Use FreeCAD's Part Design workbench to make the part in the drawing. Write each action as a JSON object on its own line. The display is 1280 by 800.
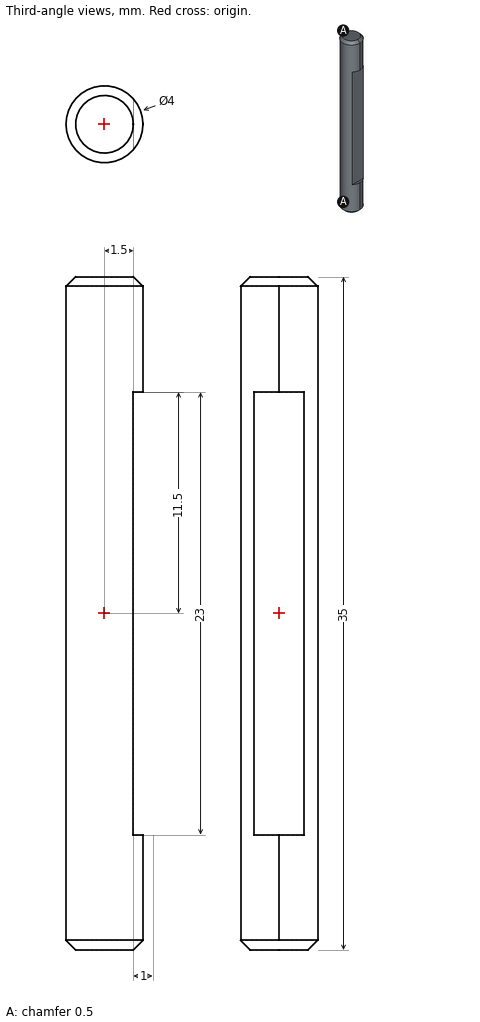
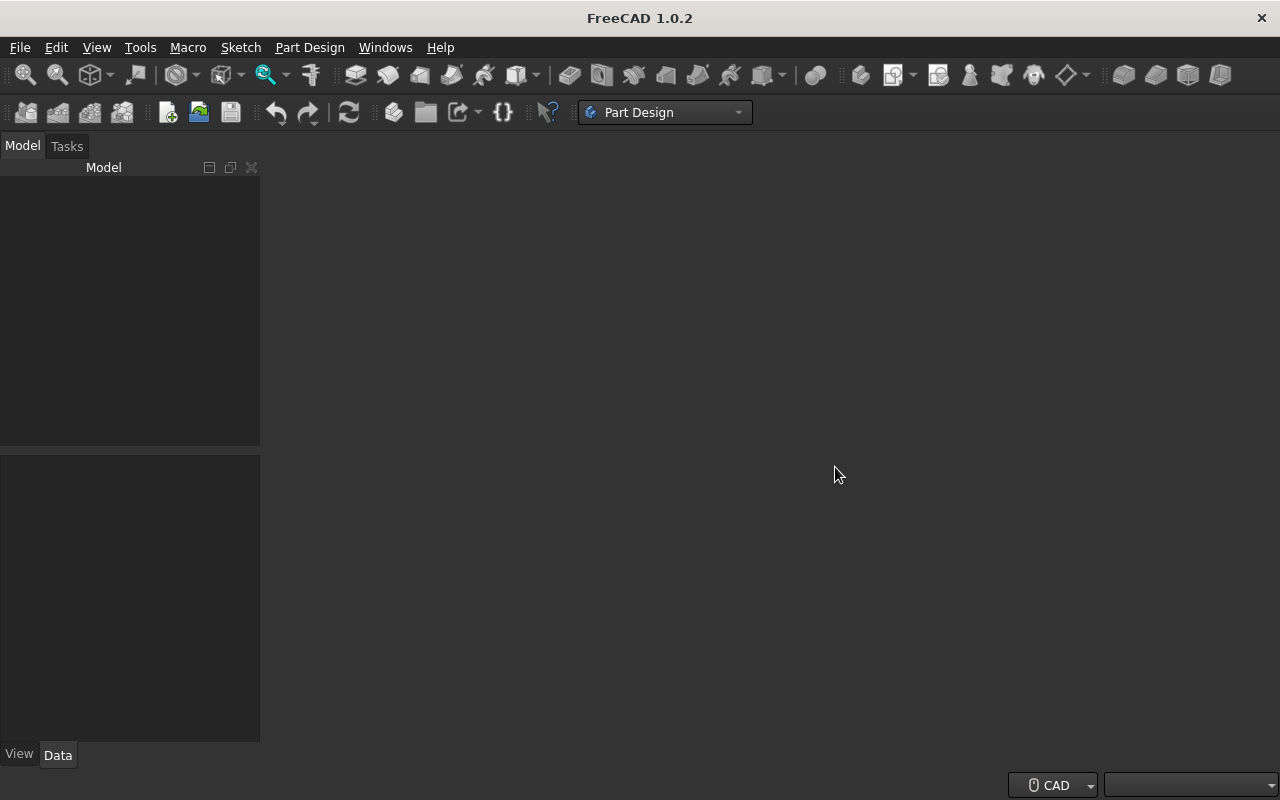
{"action": "left_click", "coordinate": [168, 112]}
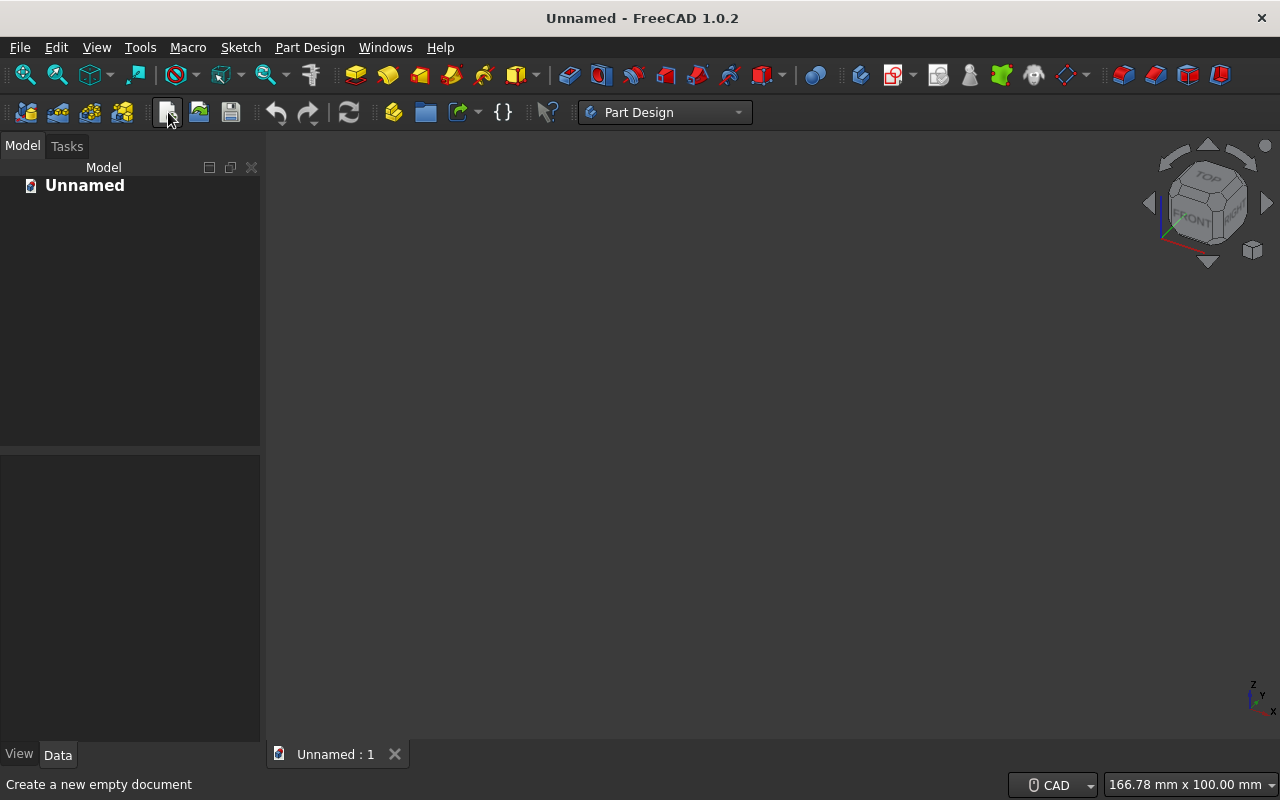
{"action": "left_click", "coordinate": [894, 76]}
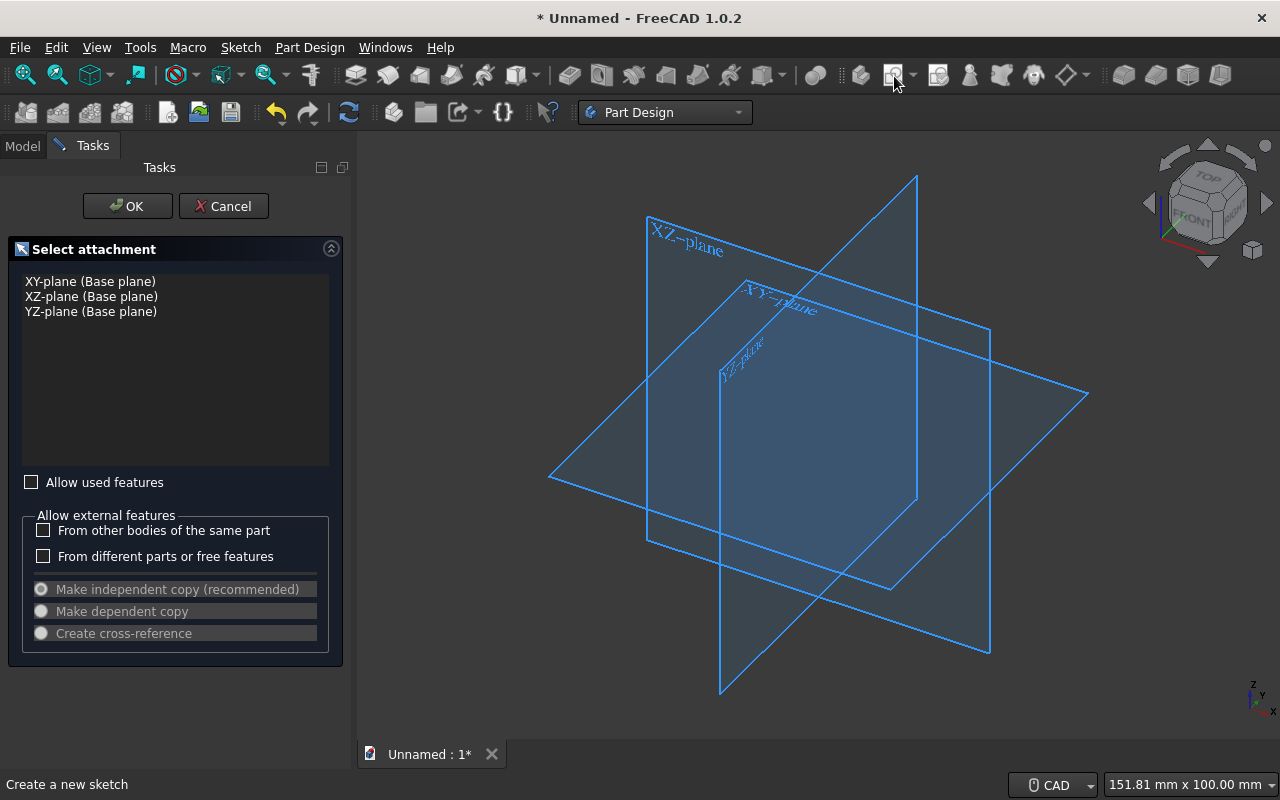
{"action": "left_click", "coordinate": [82, 282]}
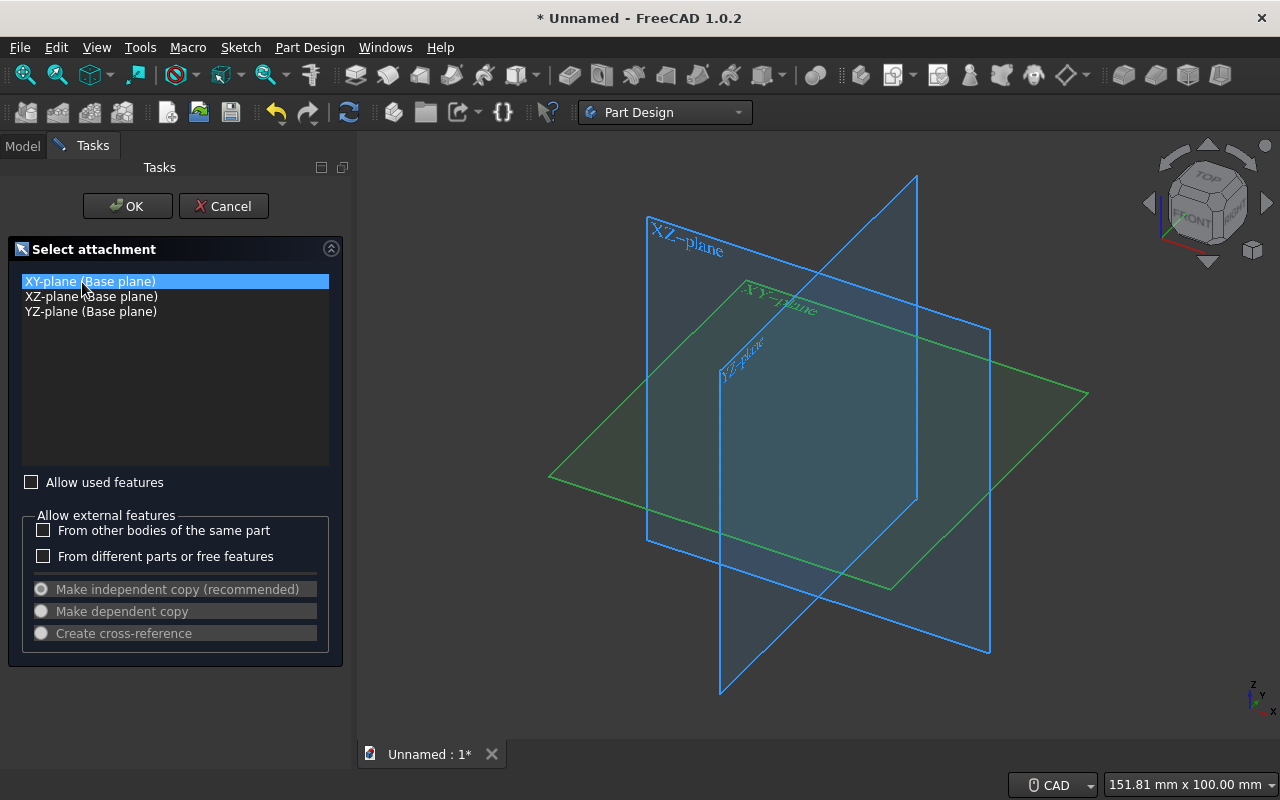
{"action": "left_click", "coordinate": [128, 206]}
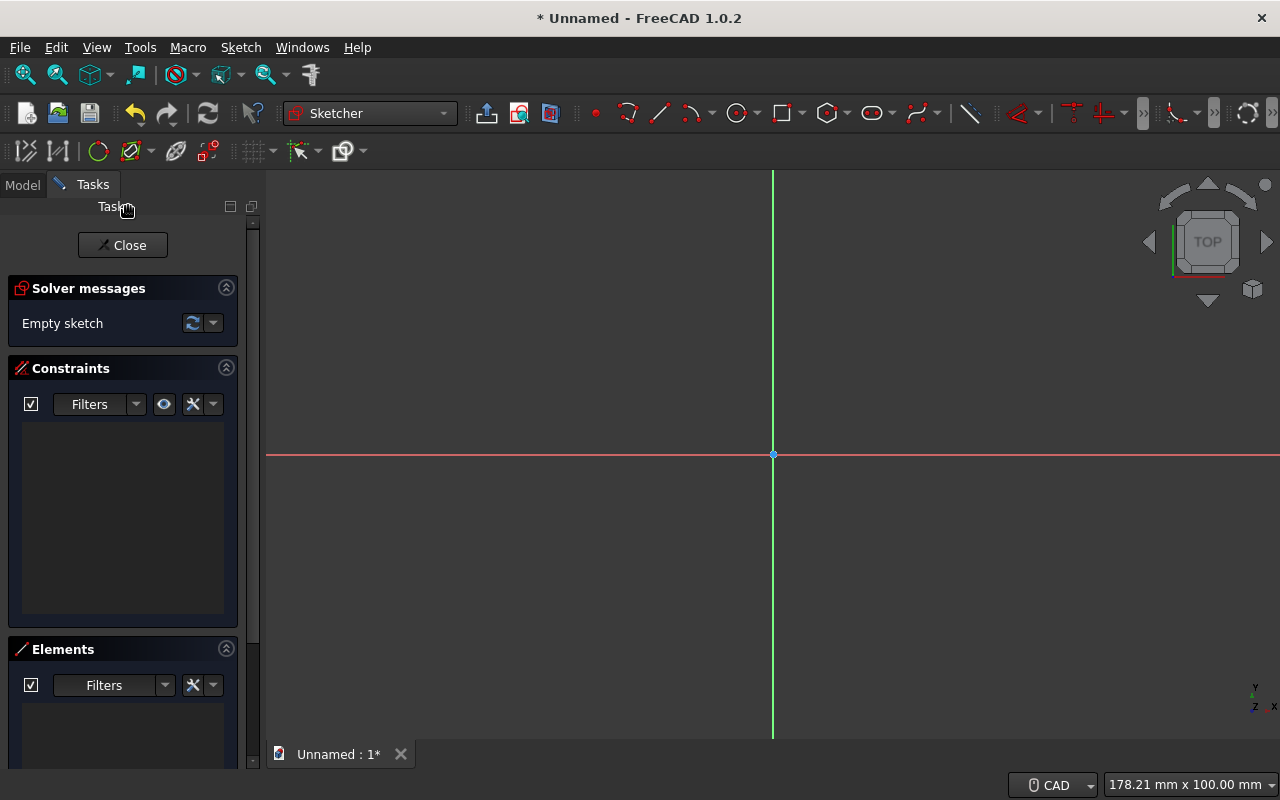
{"action": "scroll", "coordinate": [777, 454], "scroll_direction": "up", "scroll_amount": 14}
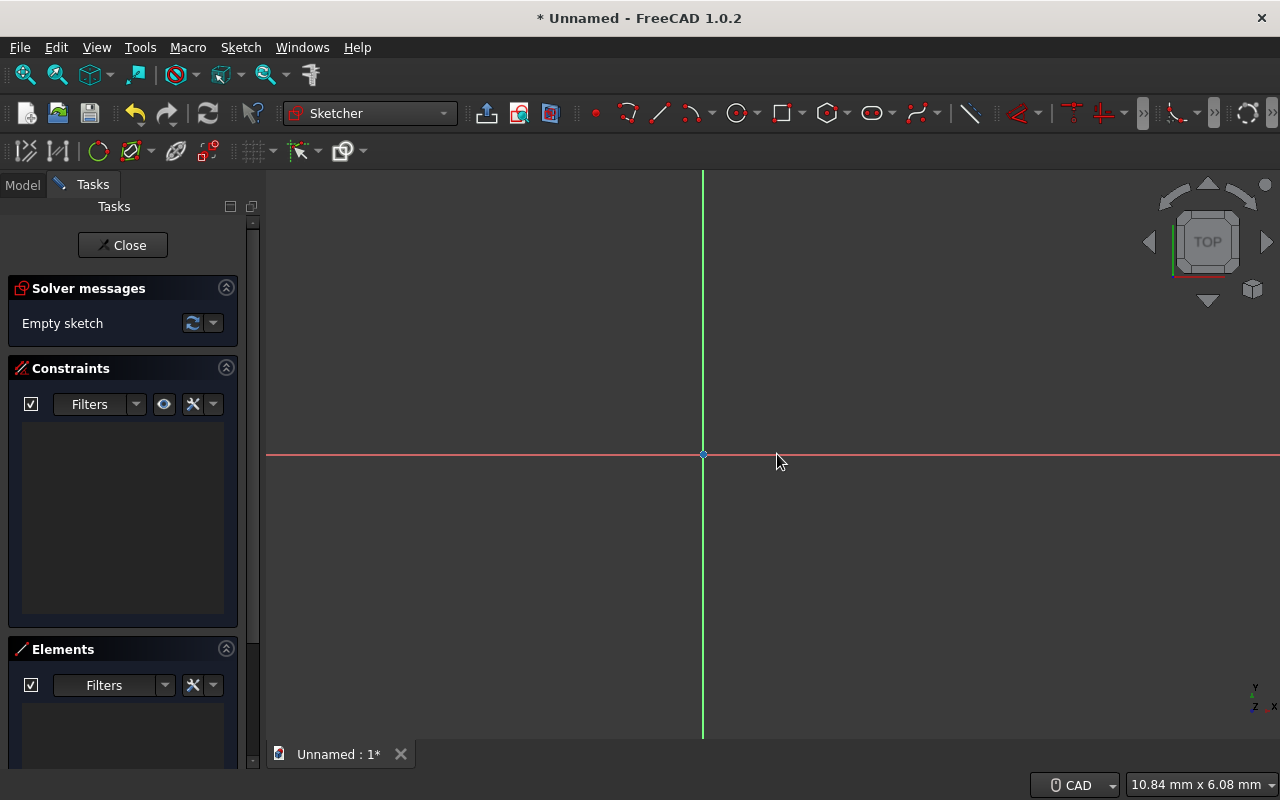
{"action": "left_click", "coordinate": [738, 114]}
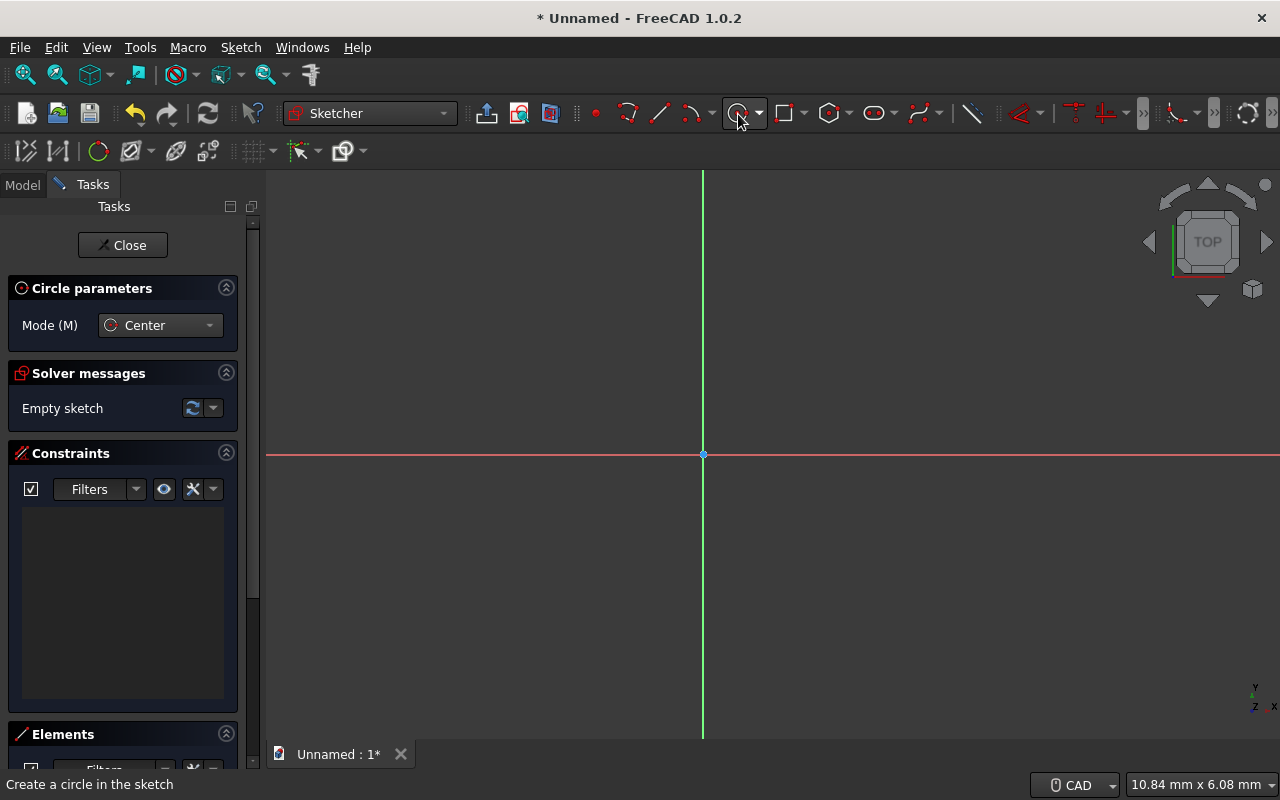
{"action": "left_click", "coordinate": [703, 454]}
{"action": "left_click", "coordinate": [836, 322]}
{"action": "key", "text": "Escape"}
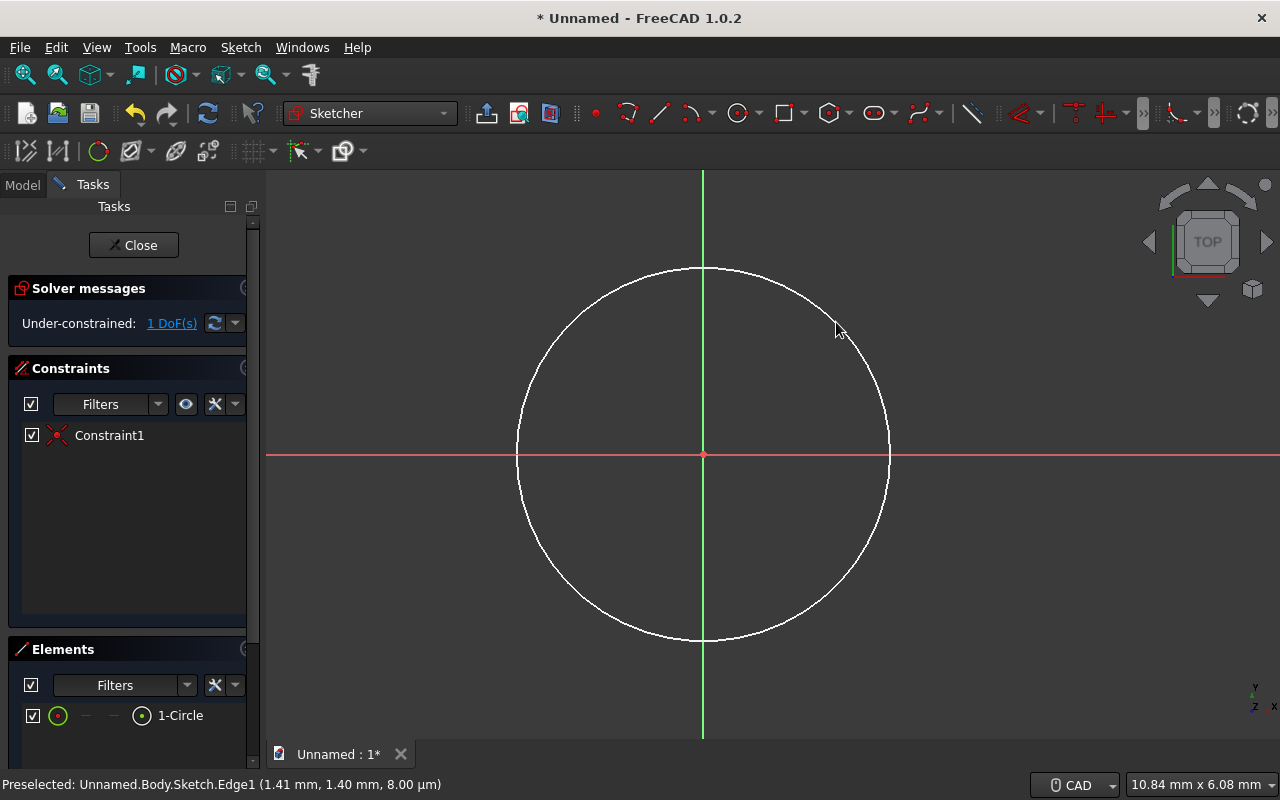
{"action": "left_click", "coordinate": [1020, 114]}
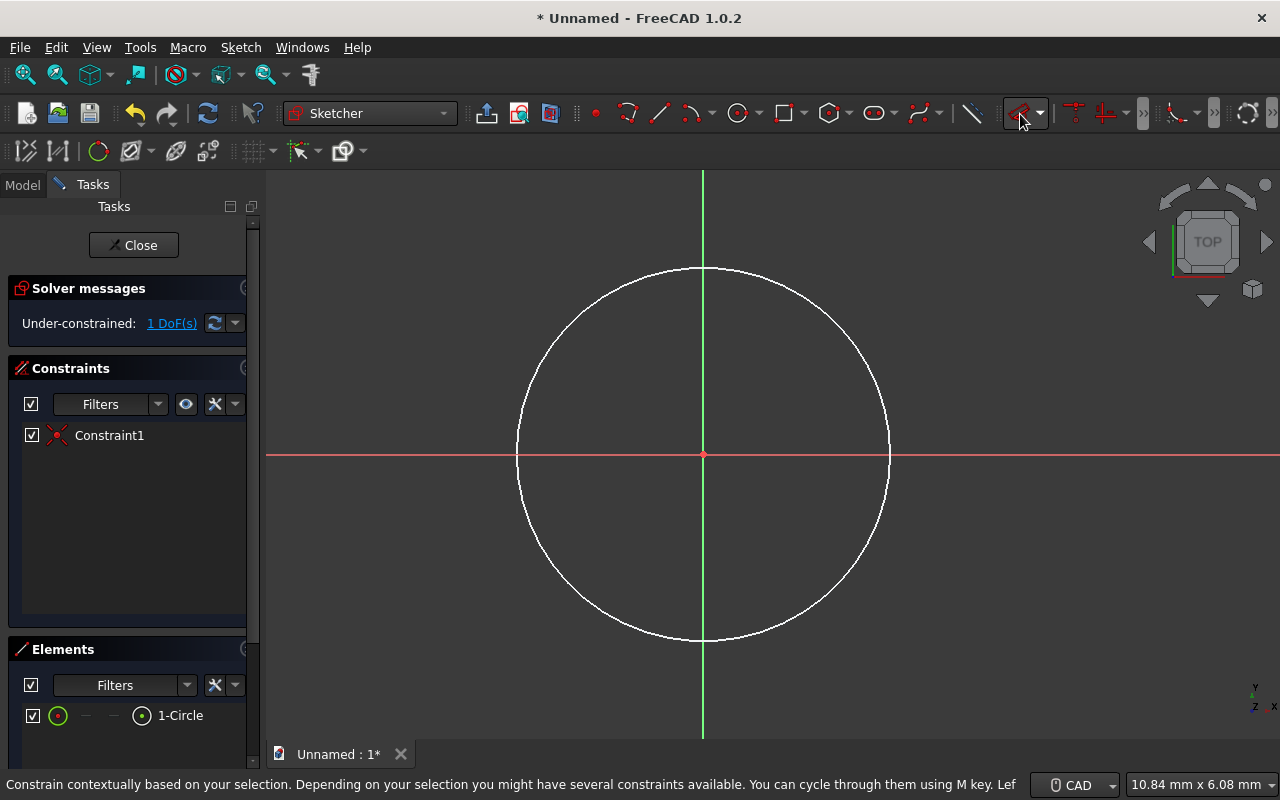
{"action": "left_click", "coordinate": [835, 322]}
{"action": "left_click", "coordinate": [858, 299]}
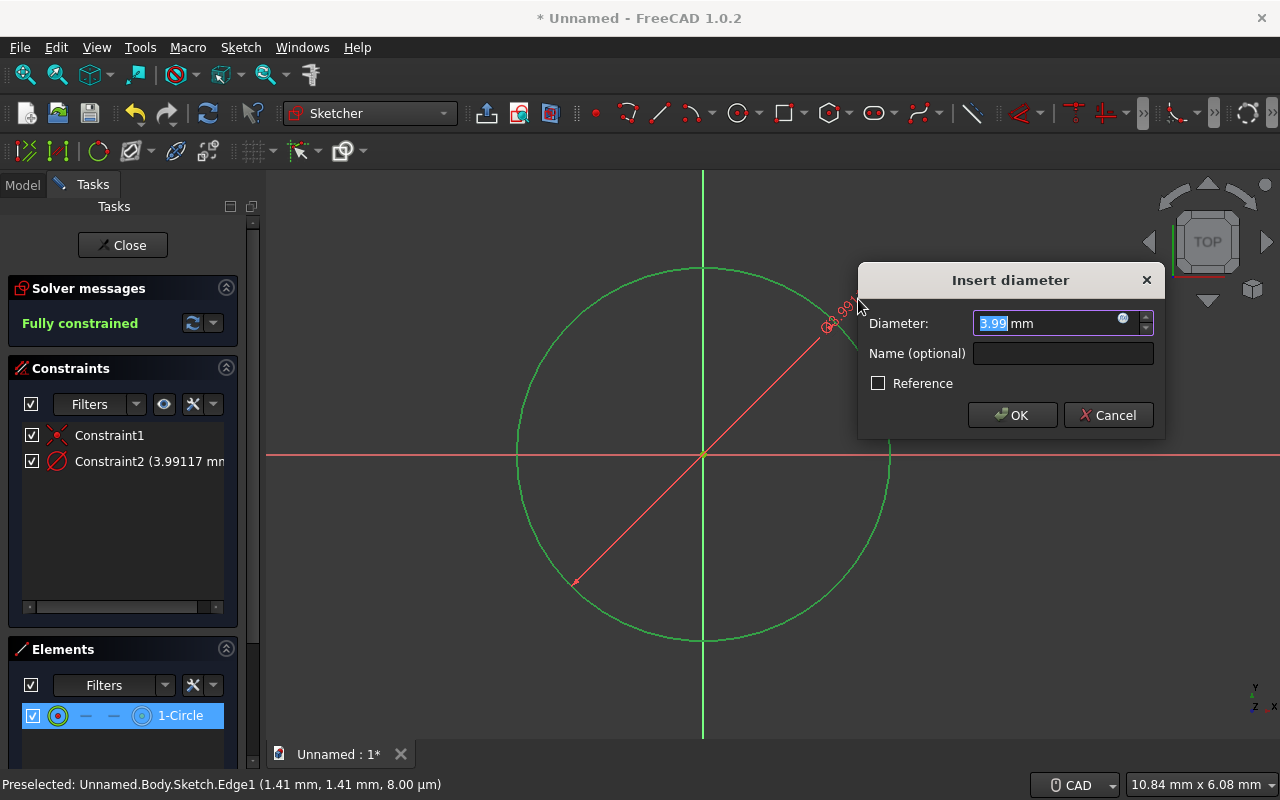
{"action": "type", "text": "4"}
{"action": "key", "text": "Return"}
{"action": "key", "text": "Escape"}